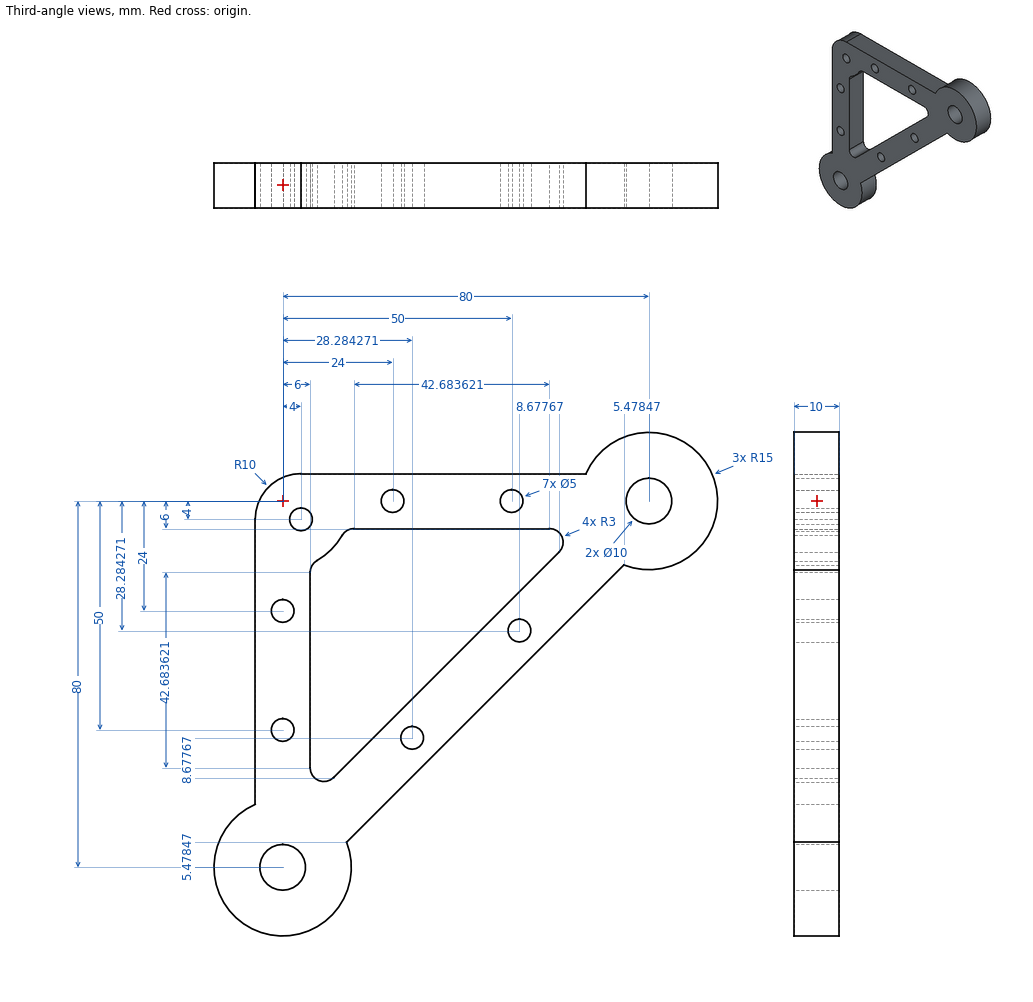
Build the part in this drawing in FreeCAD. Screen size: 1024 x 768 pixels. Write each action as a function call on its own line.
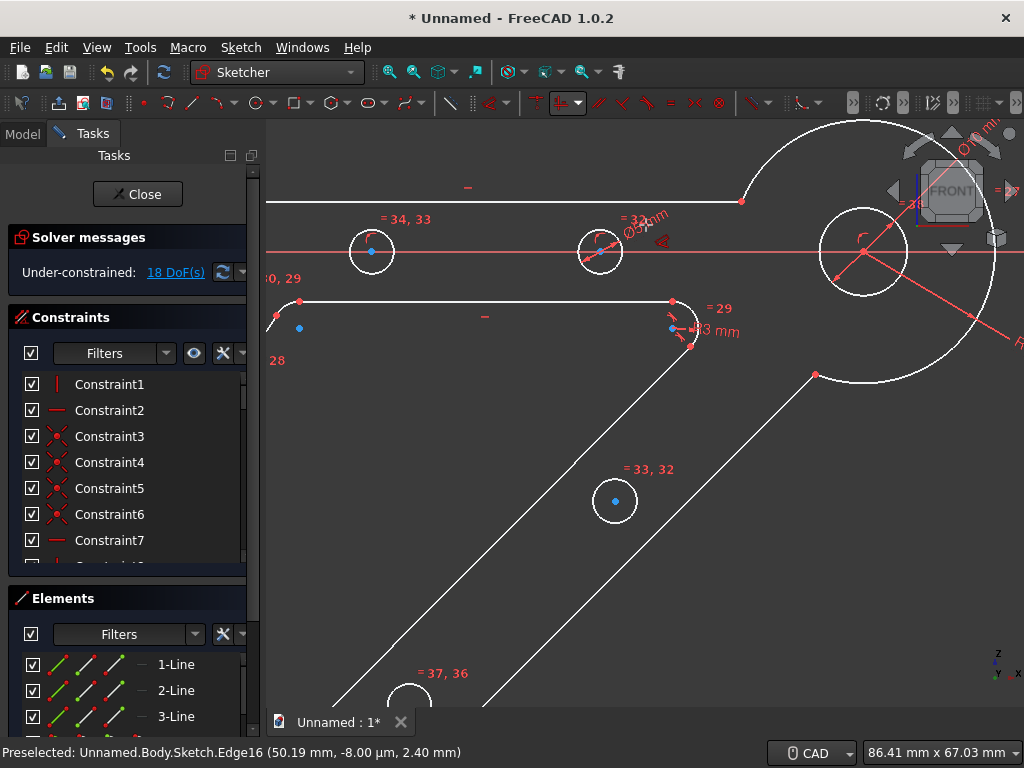
scroll(601, 230, down, 4)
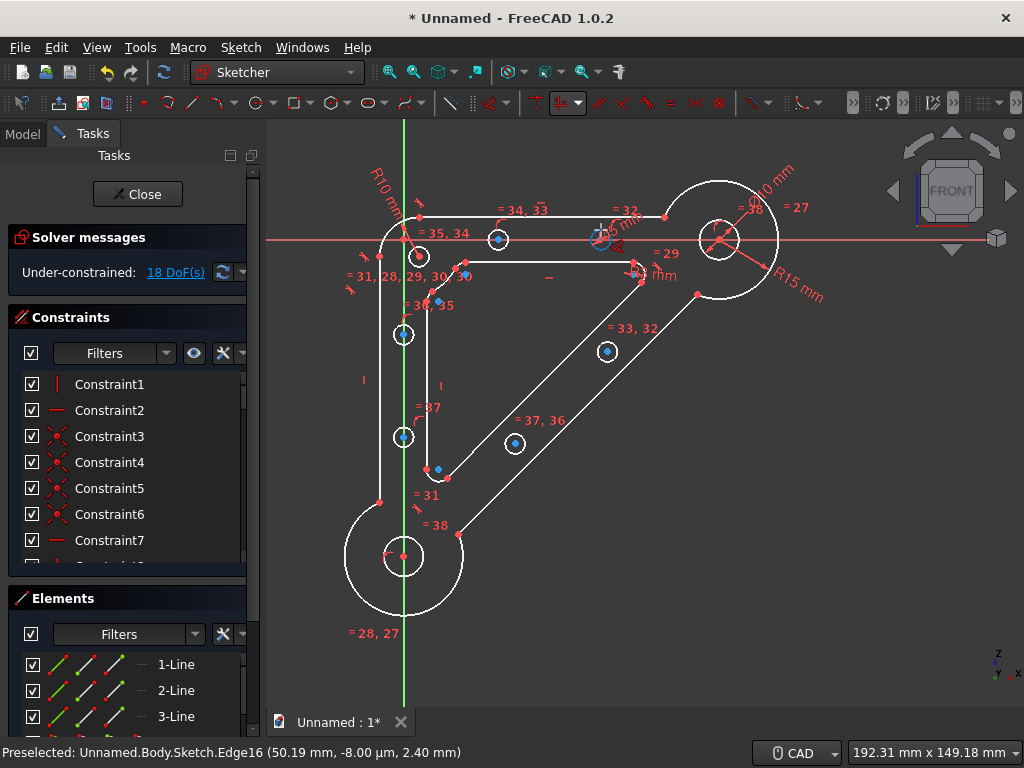
scroll(419, 257, up, 5)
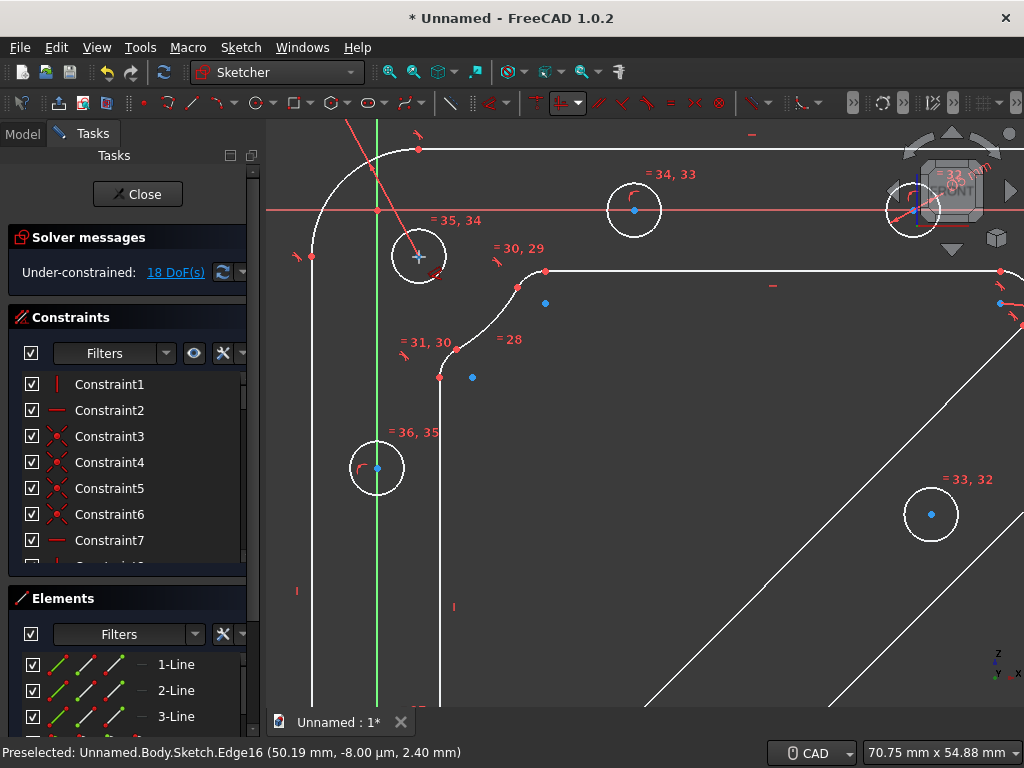
click(419, 256)
click(398, 176)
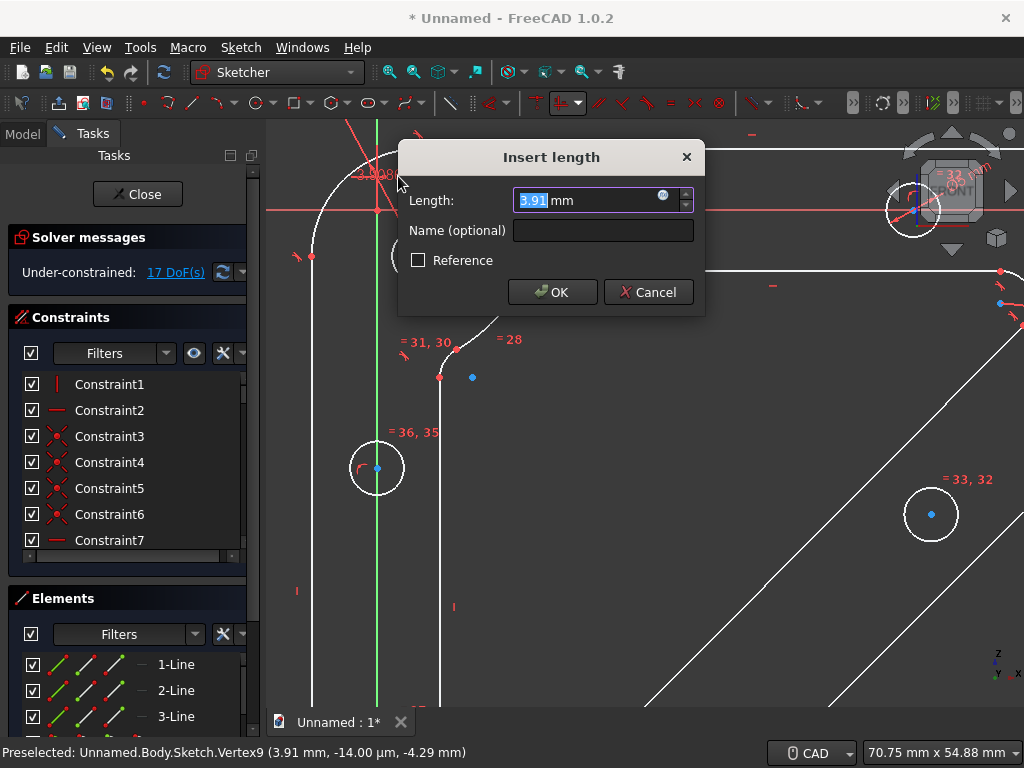
text(4)
key(Return)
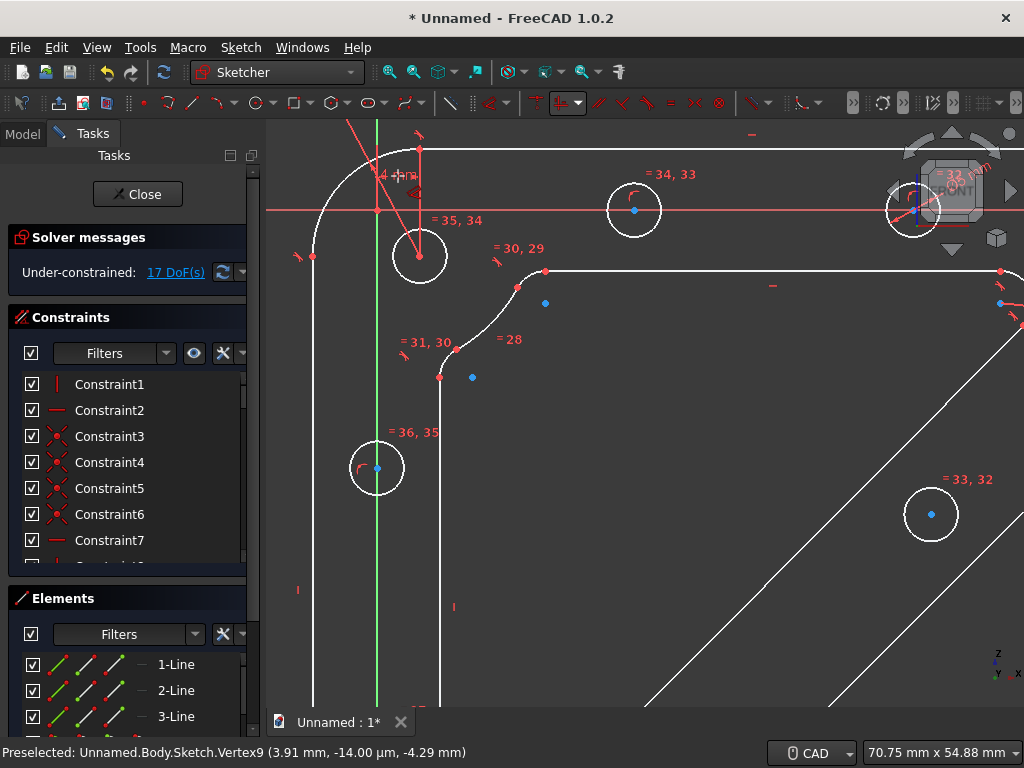
click(420, 256)
click(343, 233)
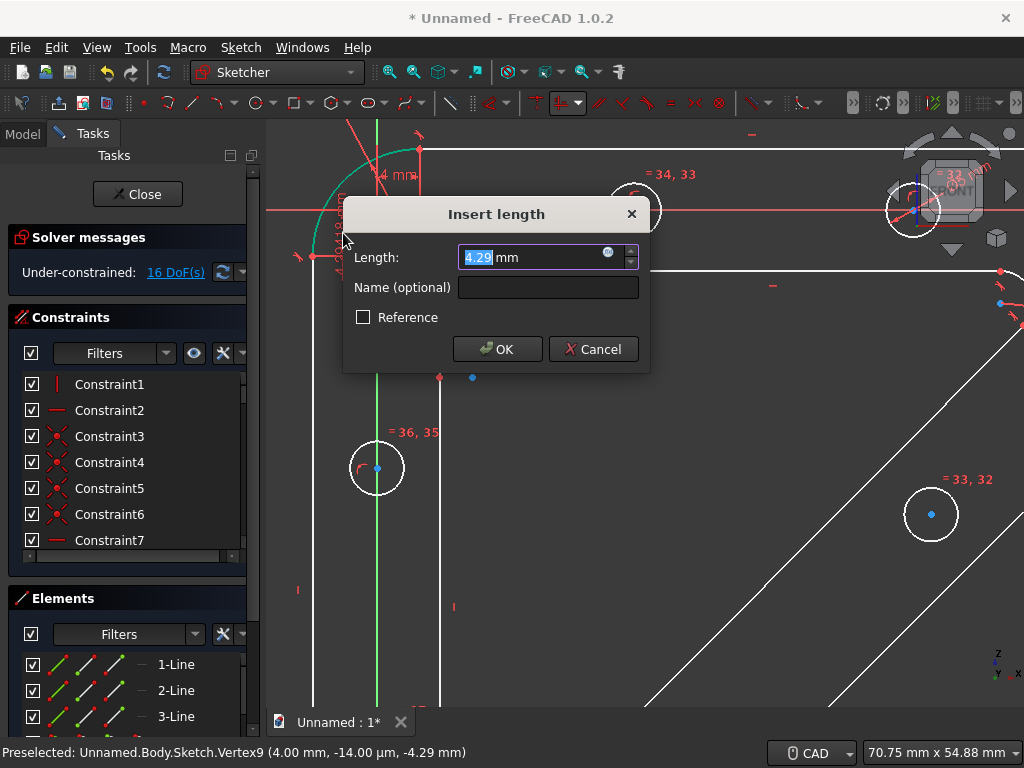
text(4)
key(Return)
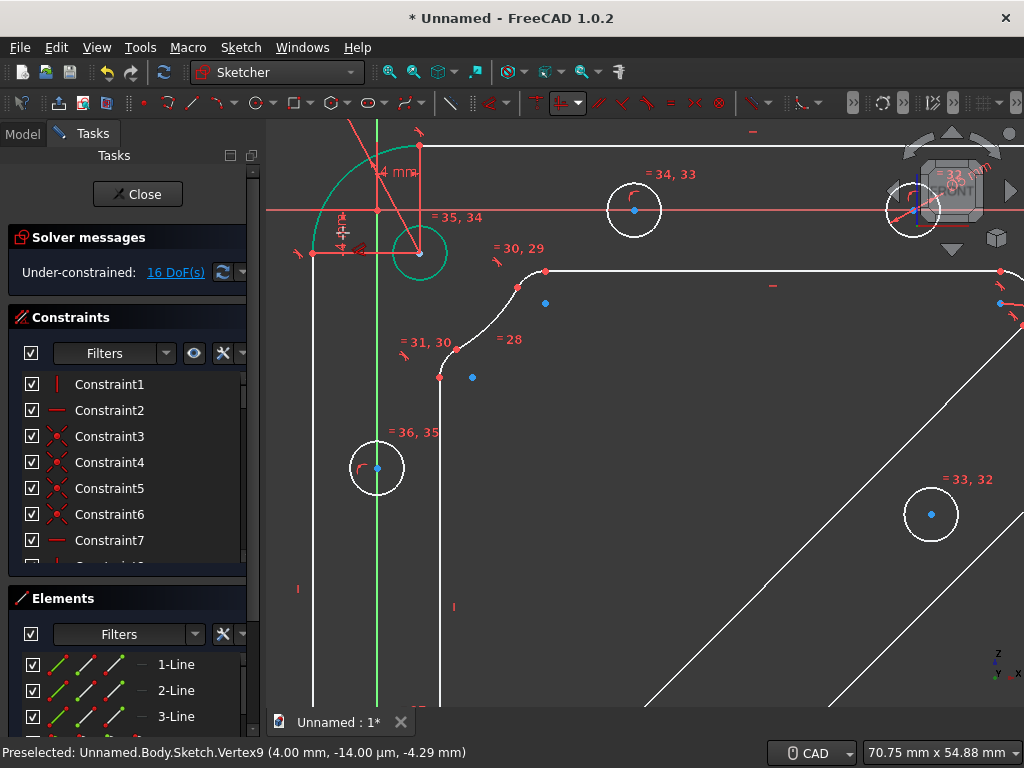
scroll(419, 257, down, 5)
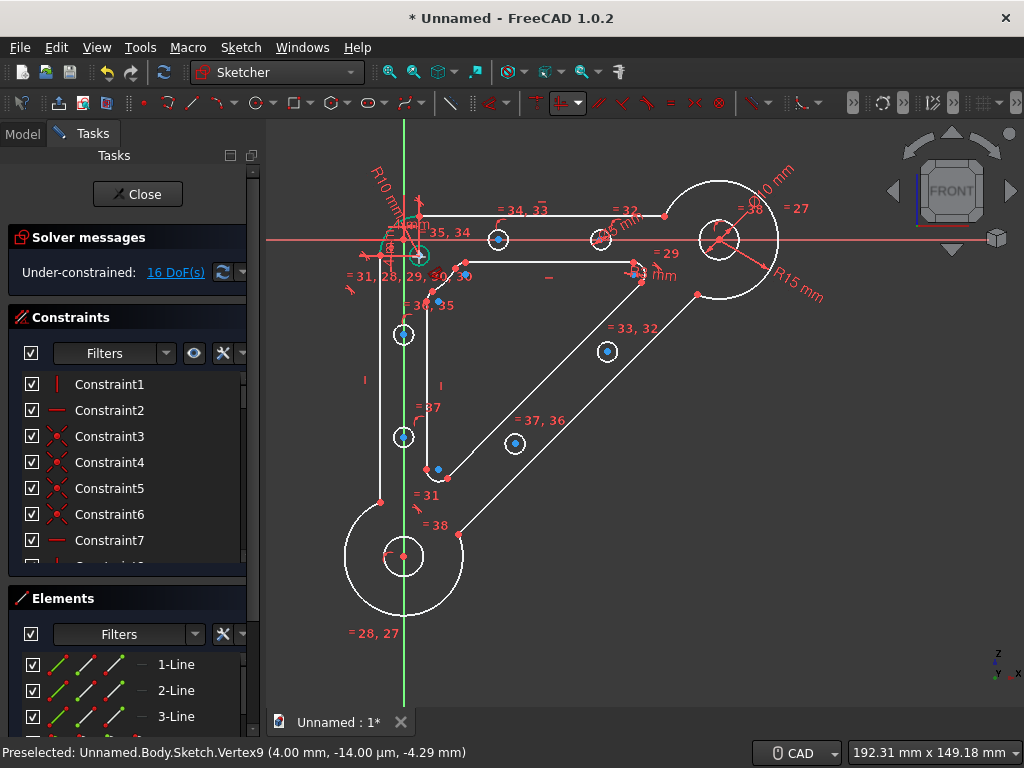
scroll(633, 262, up, 3)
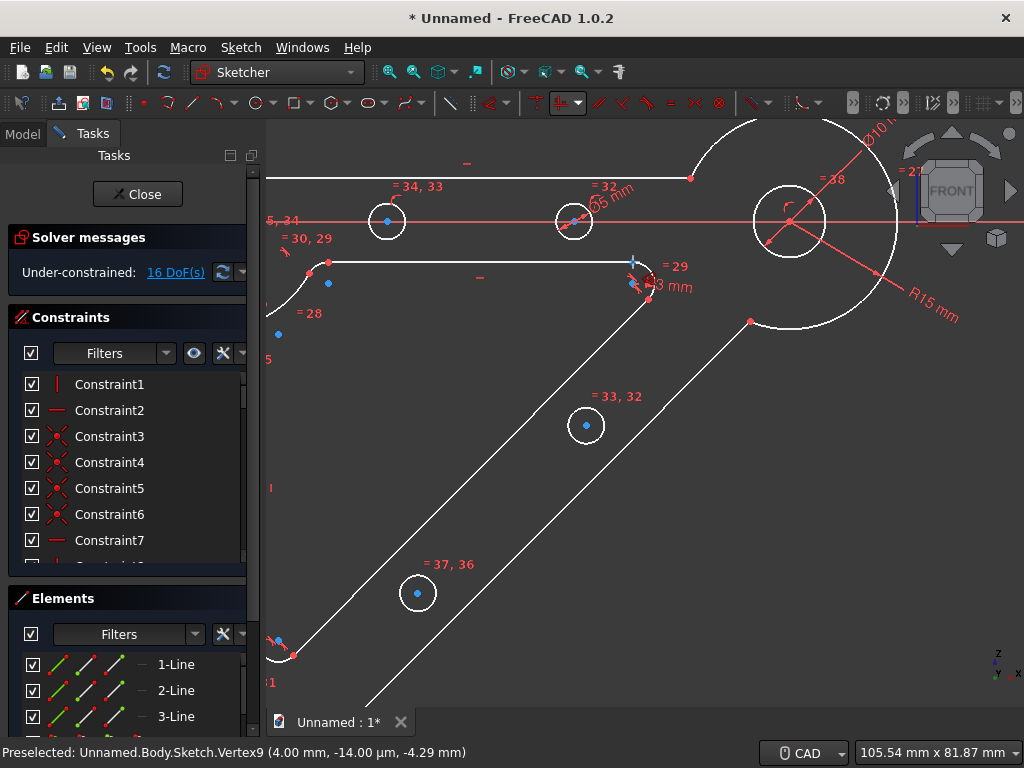
click(633, 262)
click(667, 242)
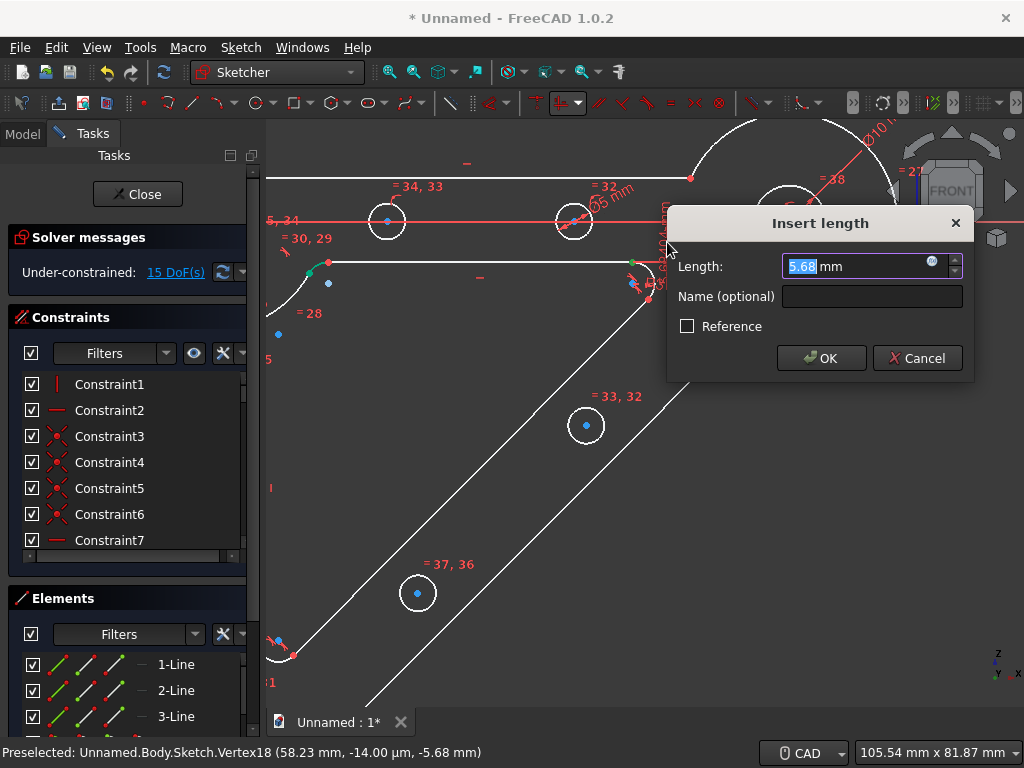
text(6)
key(Return)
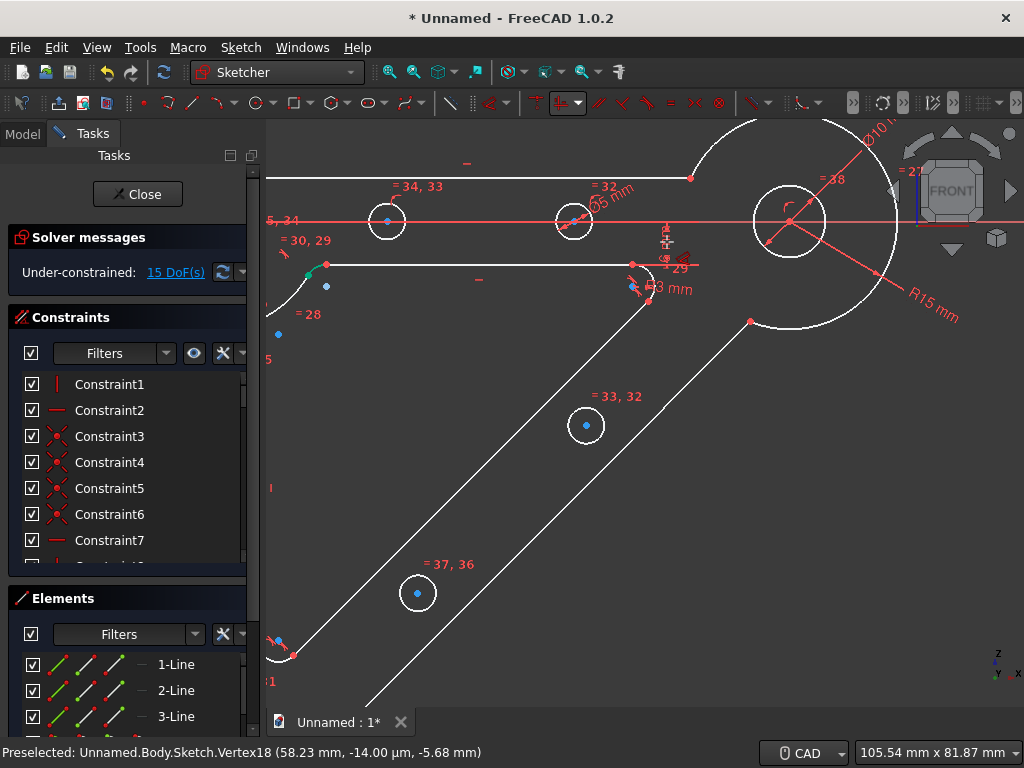
scroll(633, 262, down, 3)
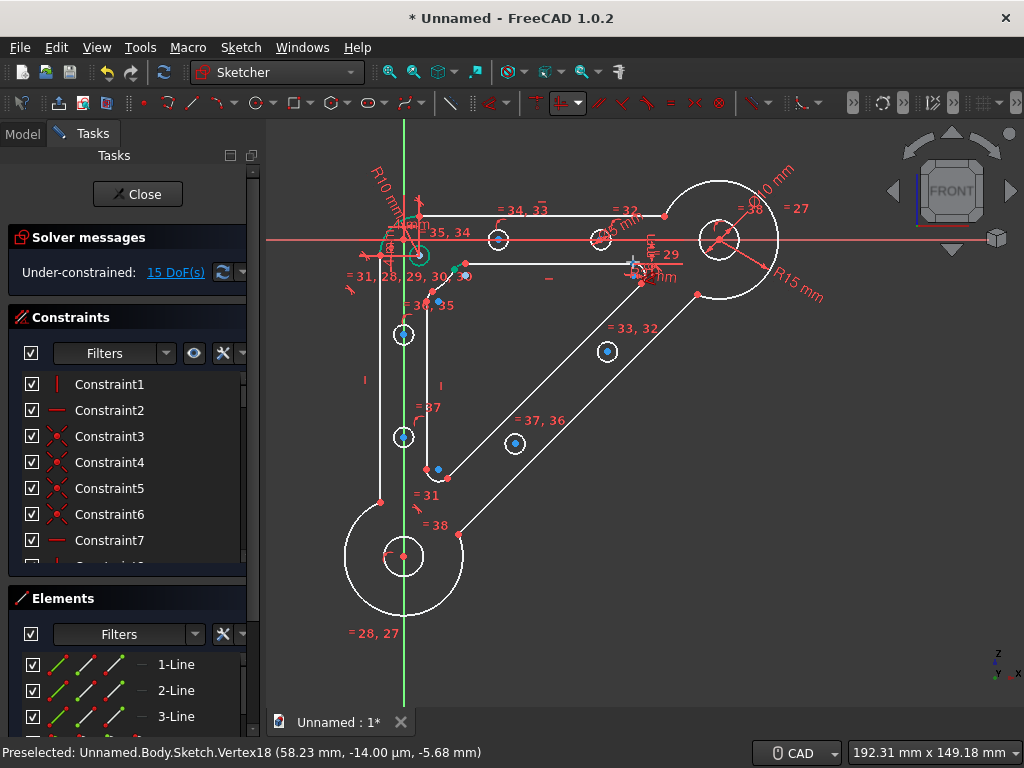
scroll(427, 302, up, 3)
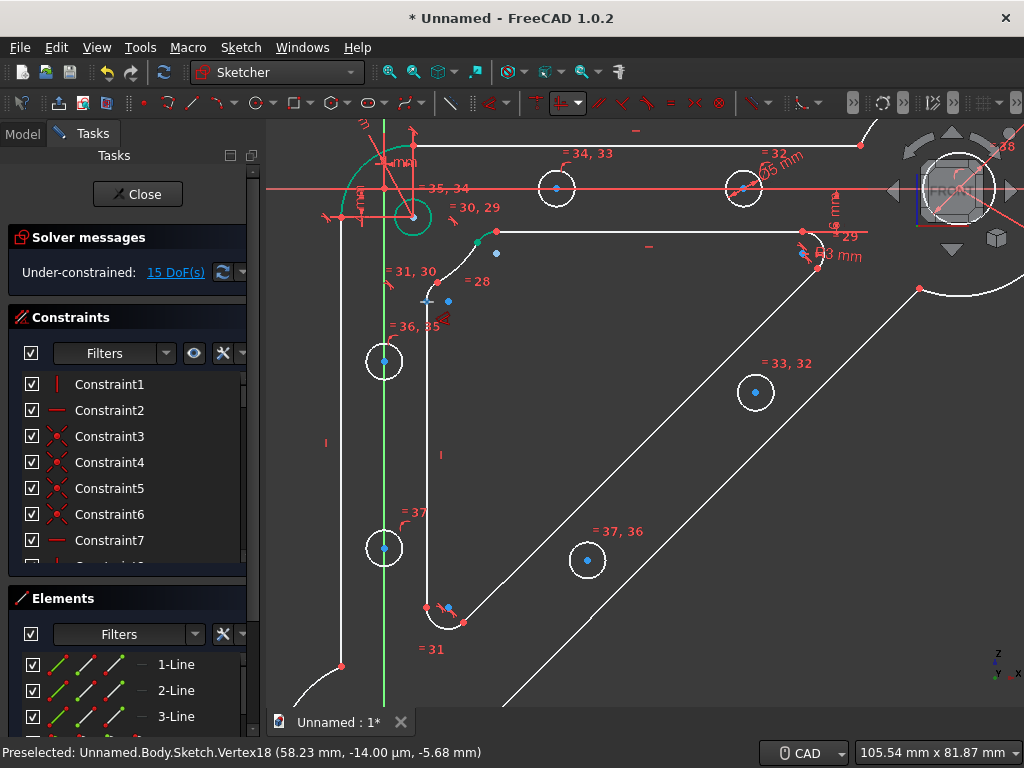
click(427, 301)
click(405, 335)